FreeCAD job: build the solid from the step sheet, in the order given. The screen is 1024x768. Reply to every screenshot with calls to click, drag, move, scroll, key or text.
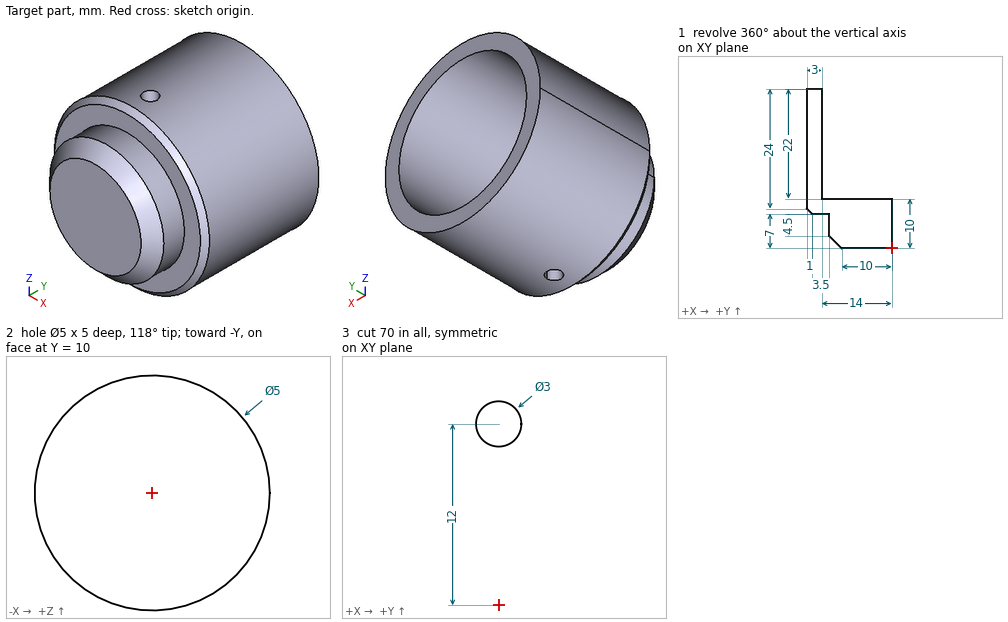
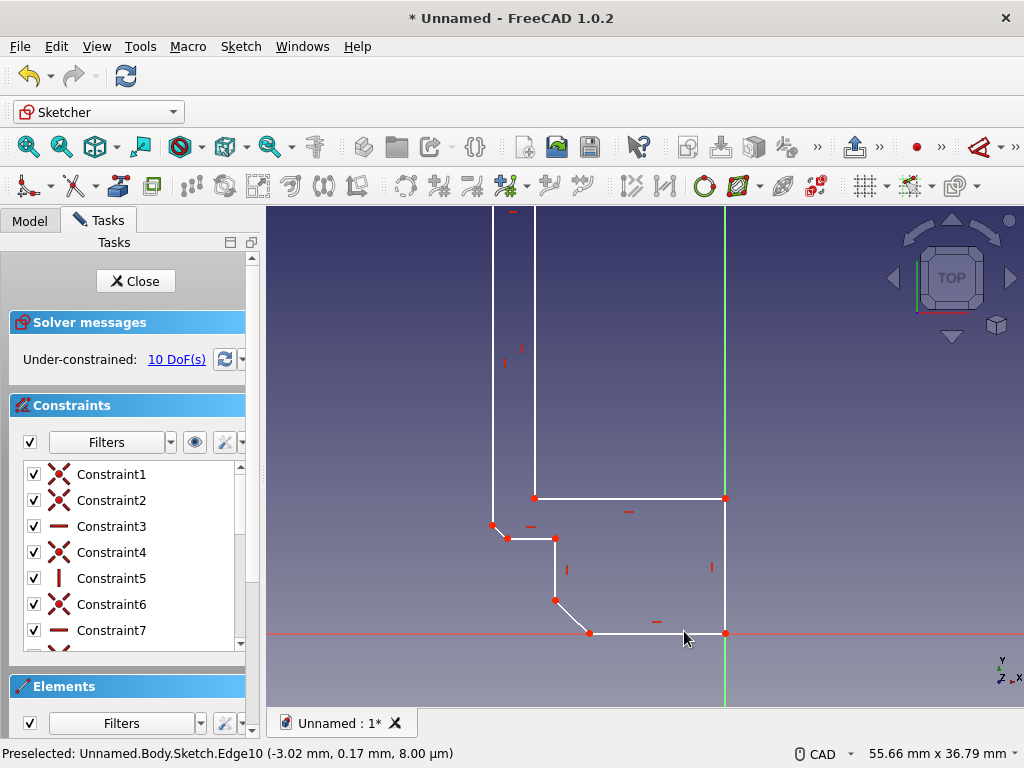
click(978, 148)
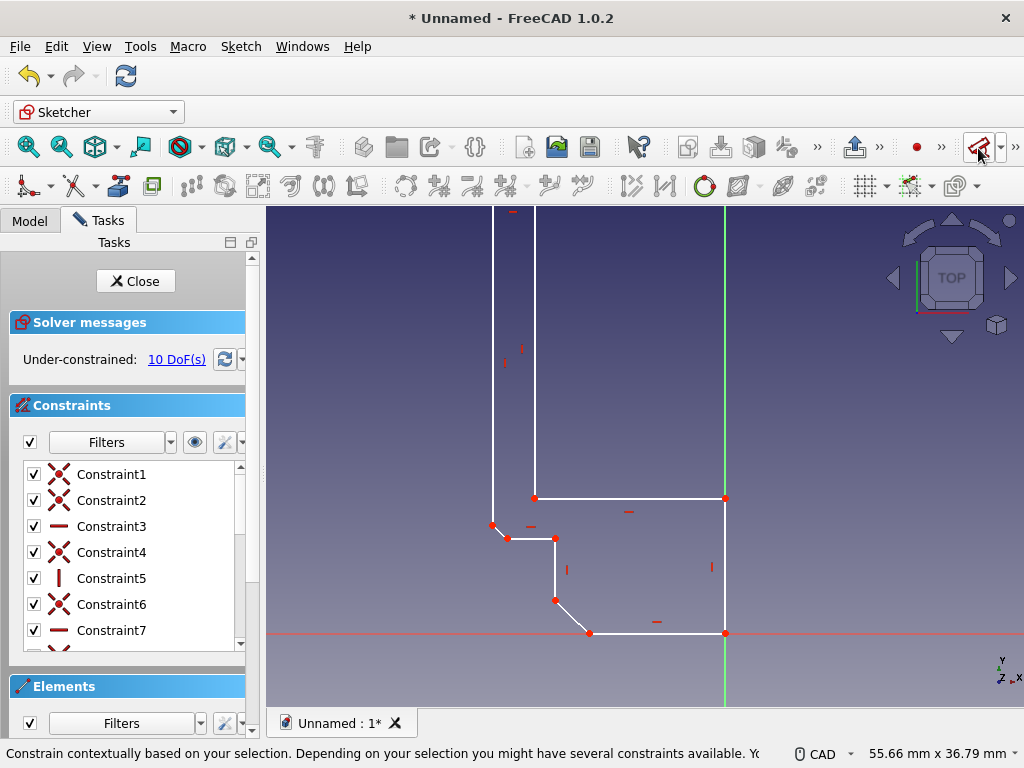
scroll(510, 539, down, 2)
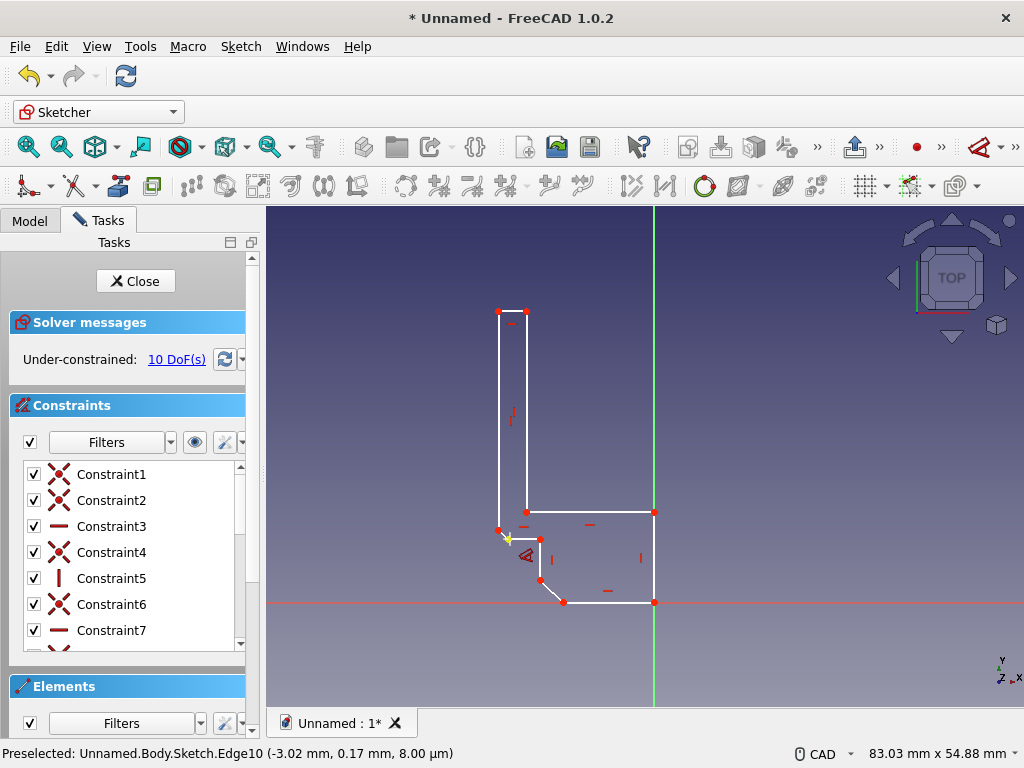
scroll(518, 311, up, 3)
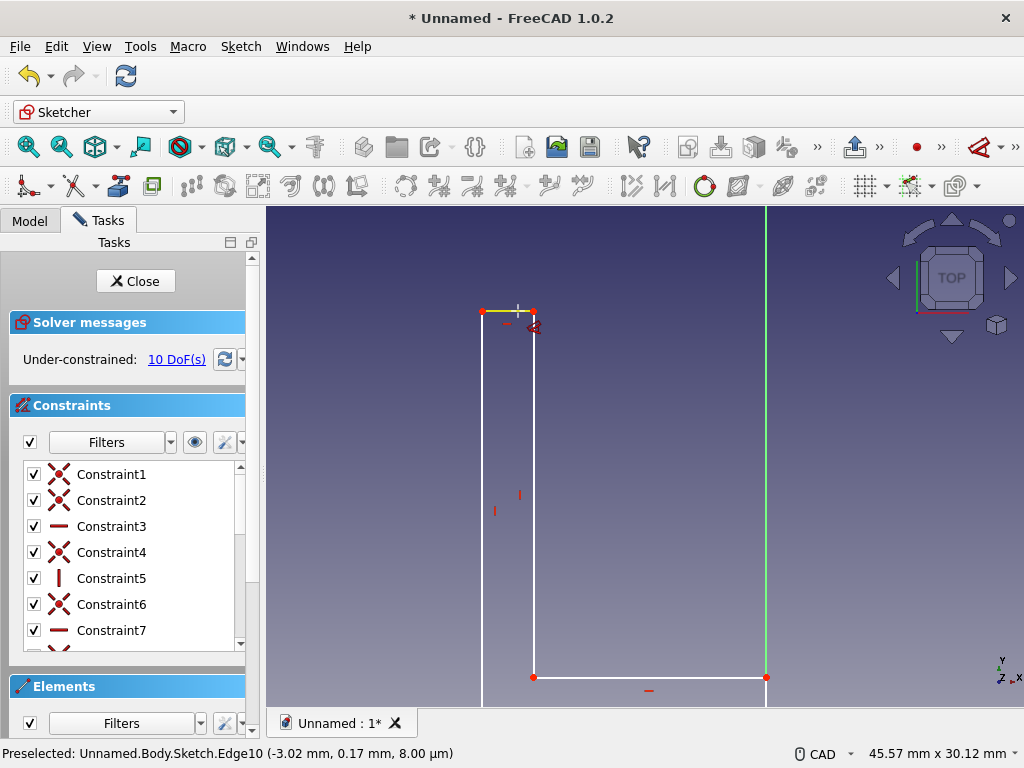
click(518, 311)
click(508, 277)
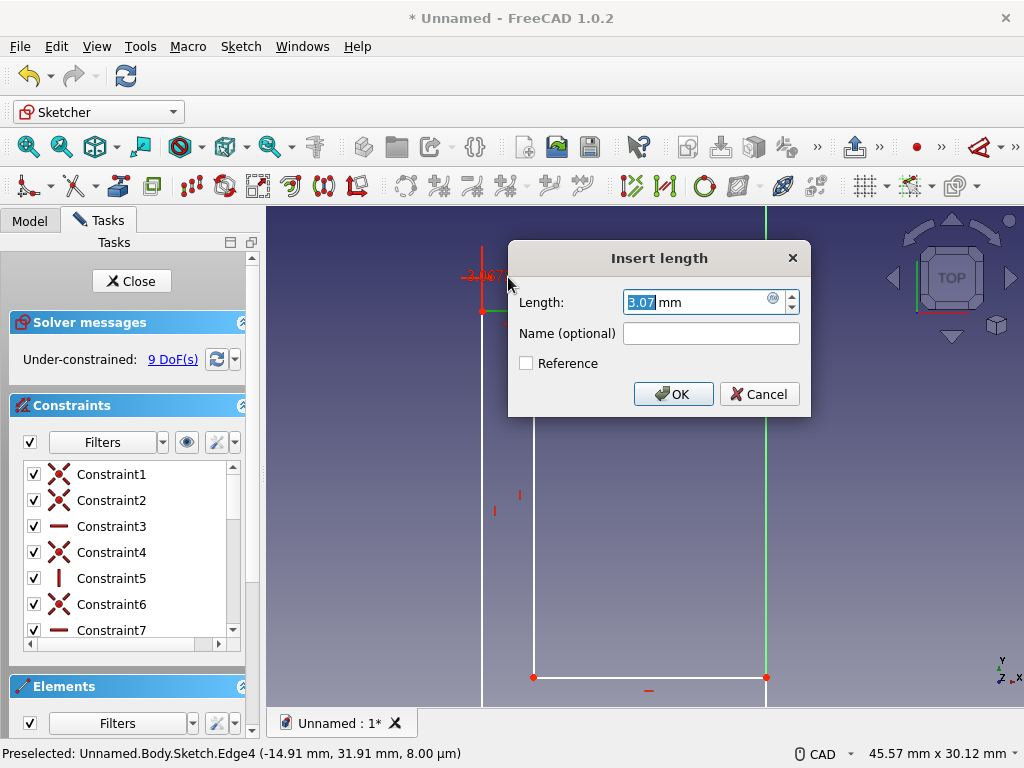
text(3)
key(Return)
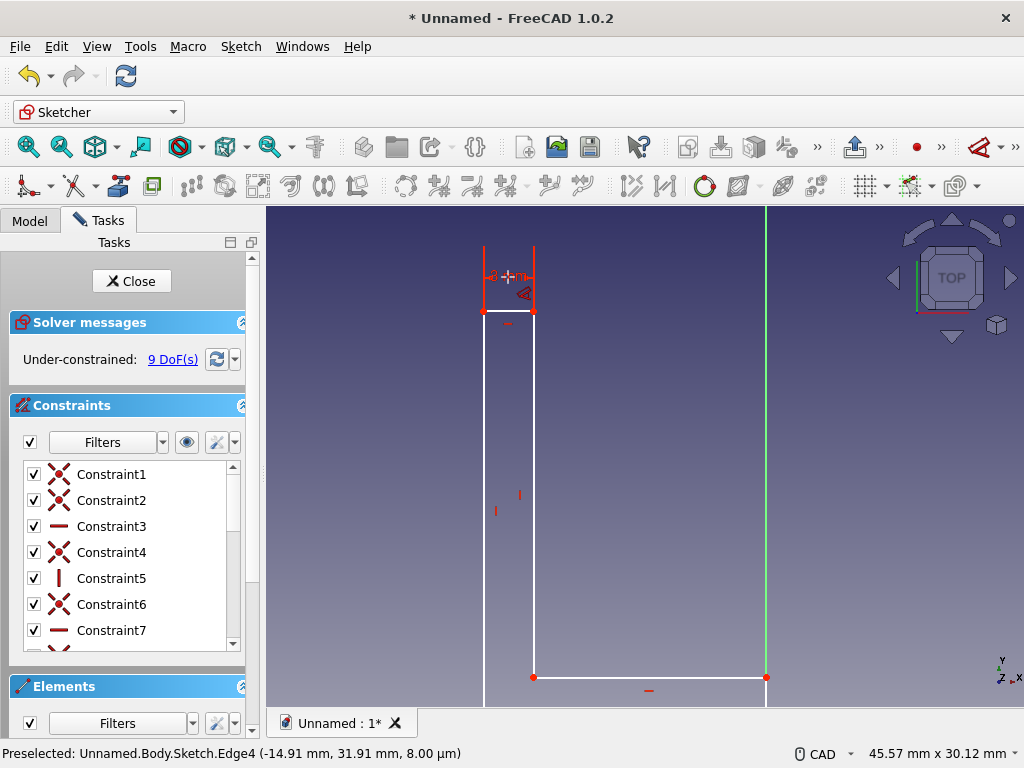
scroll(518, 311, down, 3)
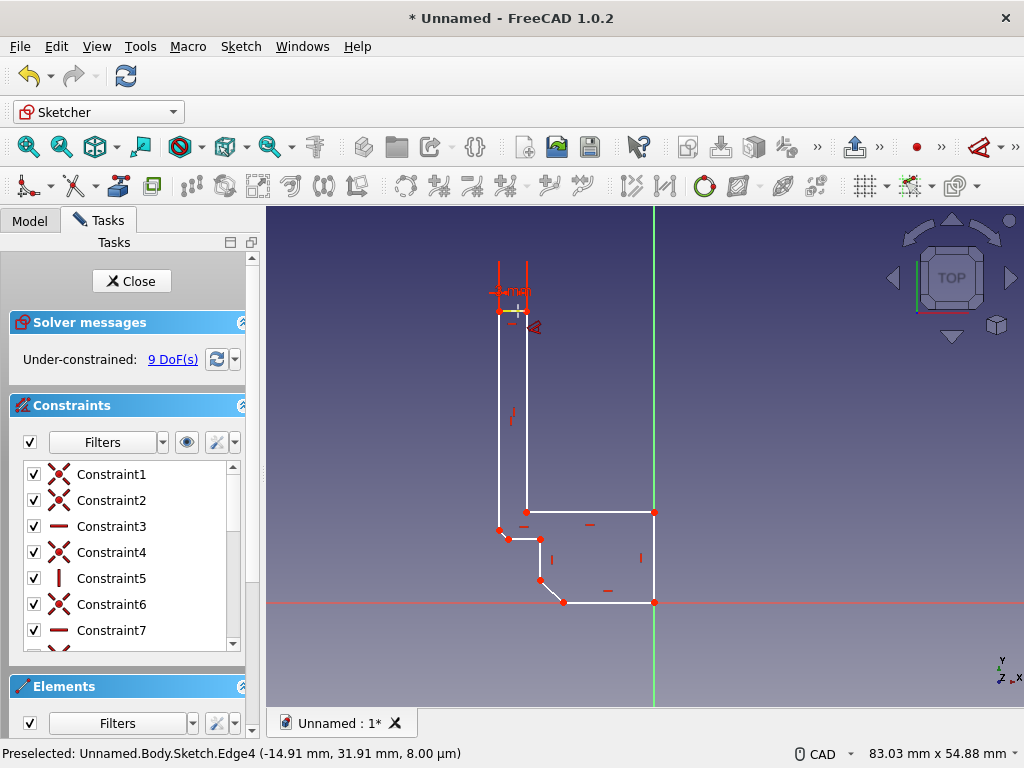
click(654, 576)
click(688, 557)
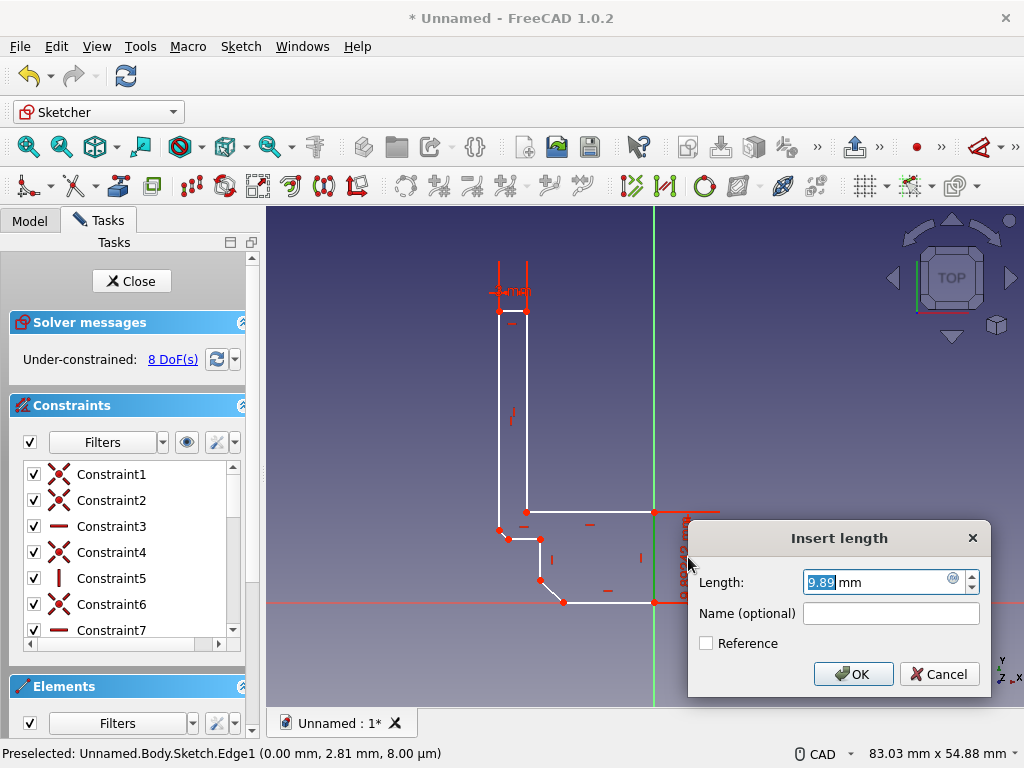
text(10)
key(Return)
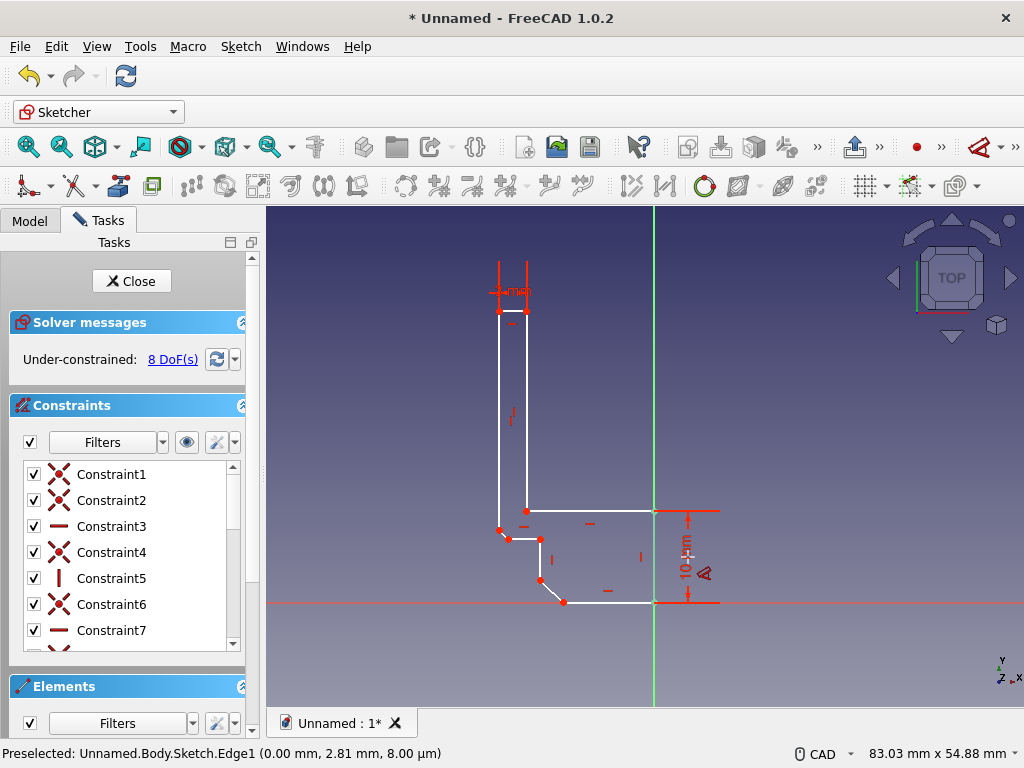
click(616, 511)
click(590, 545)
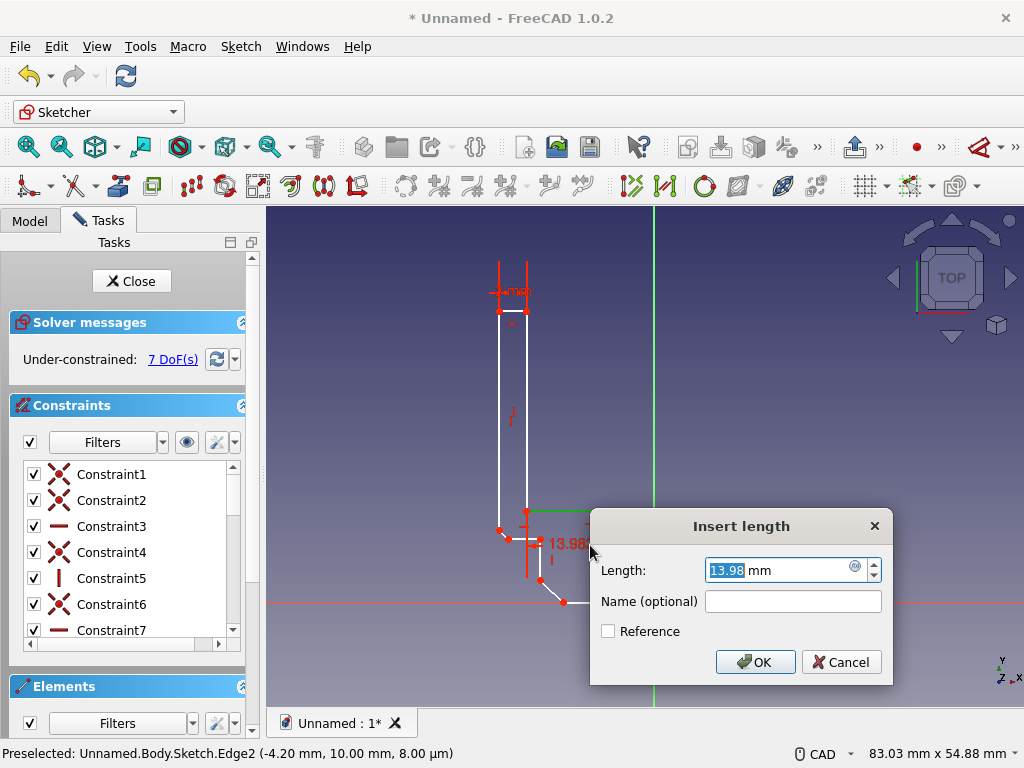
text(14)
key(Return)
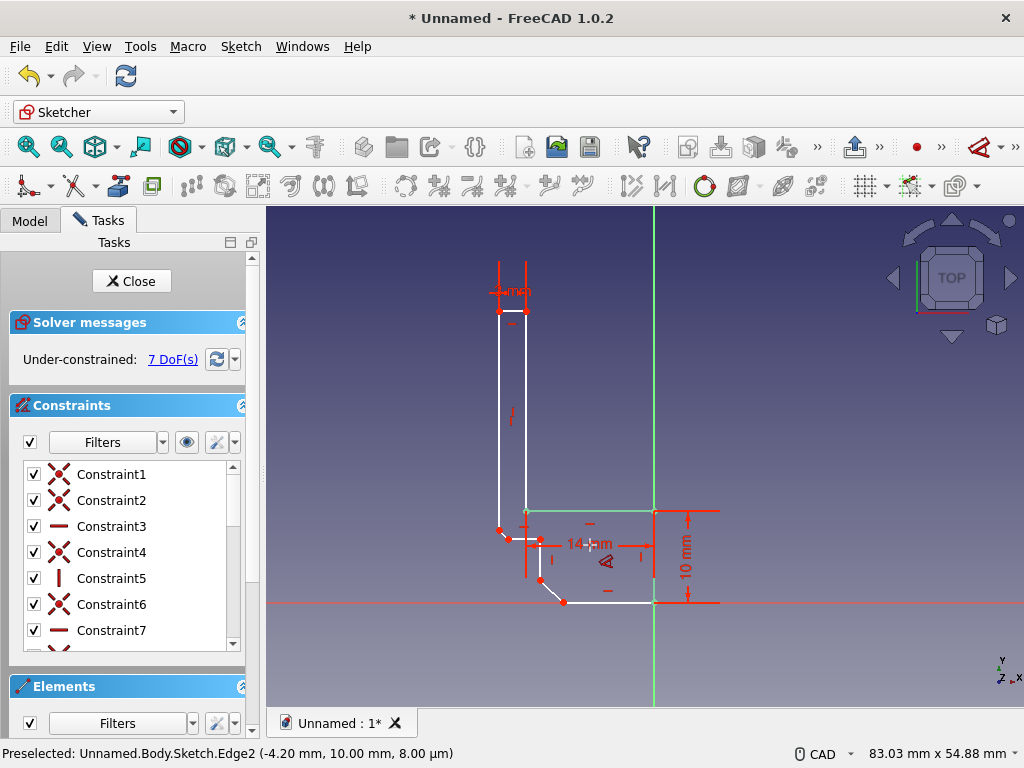
click(527, 451)
click(561, 411)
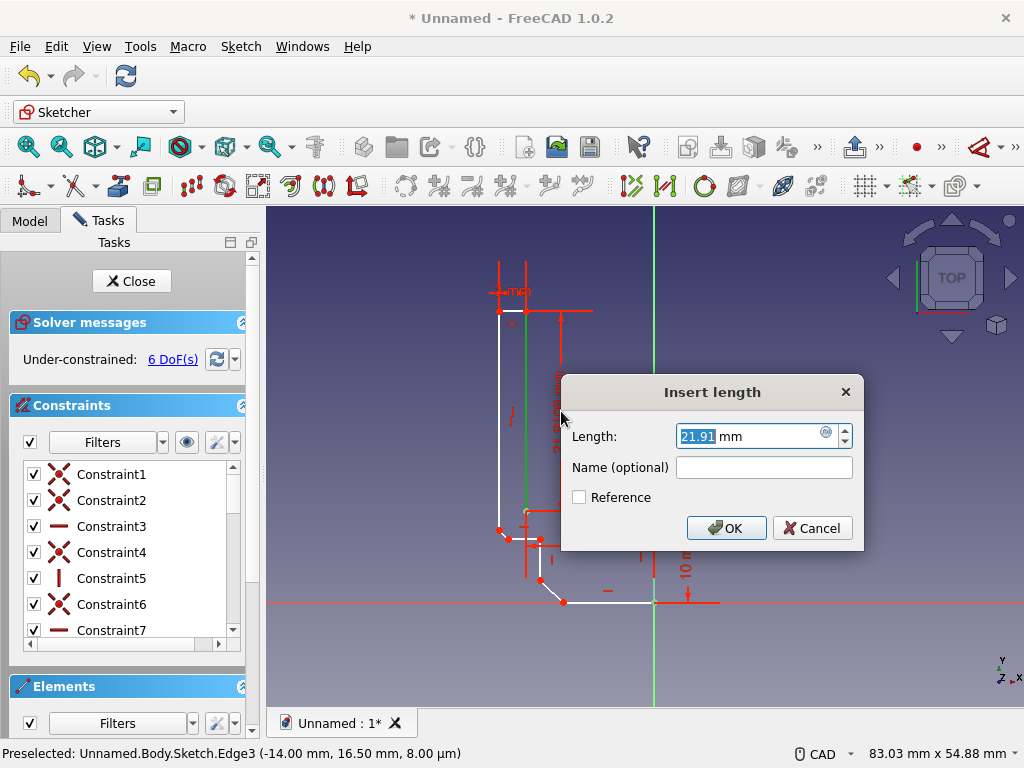
text(22)
key(Return)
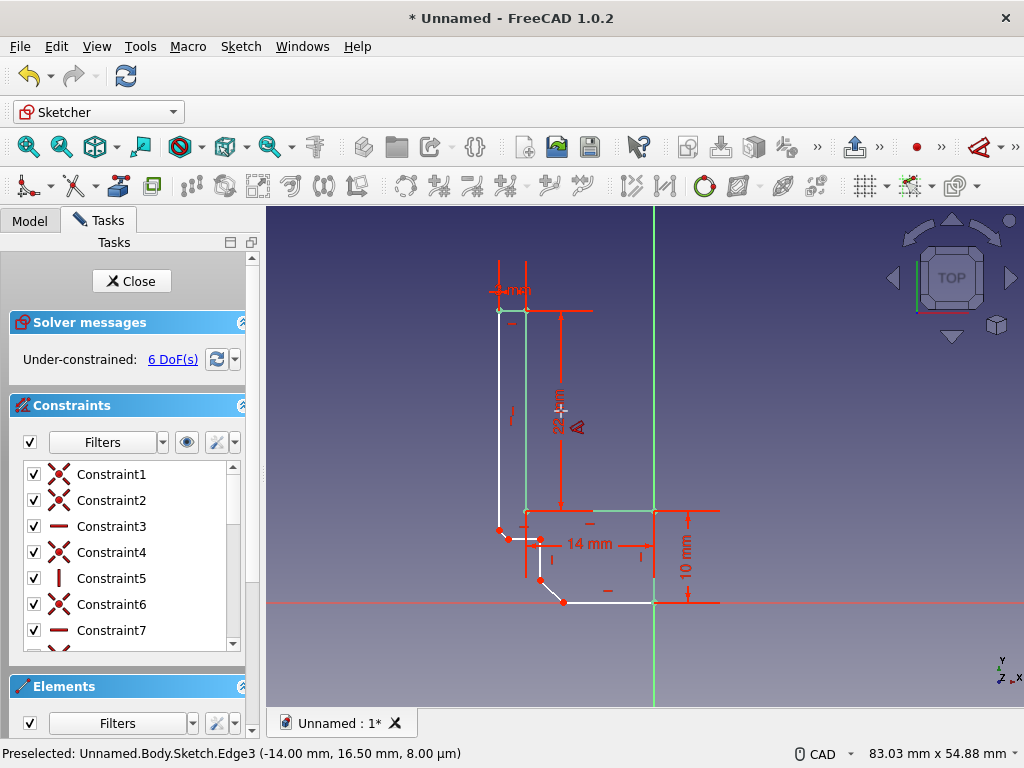
click(499, 376)
click(465, 420)